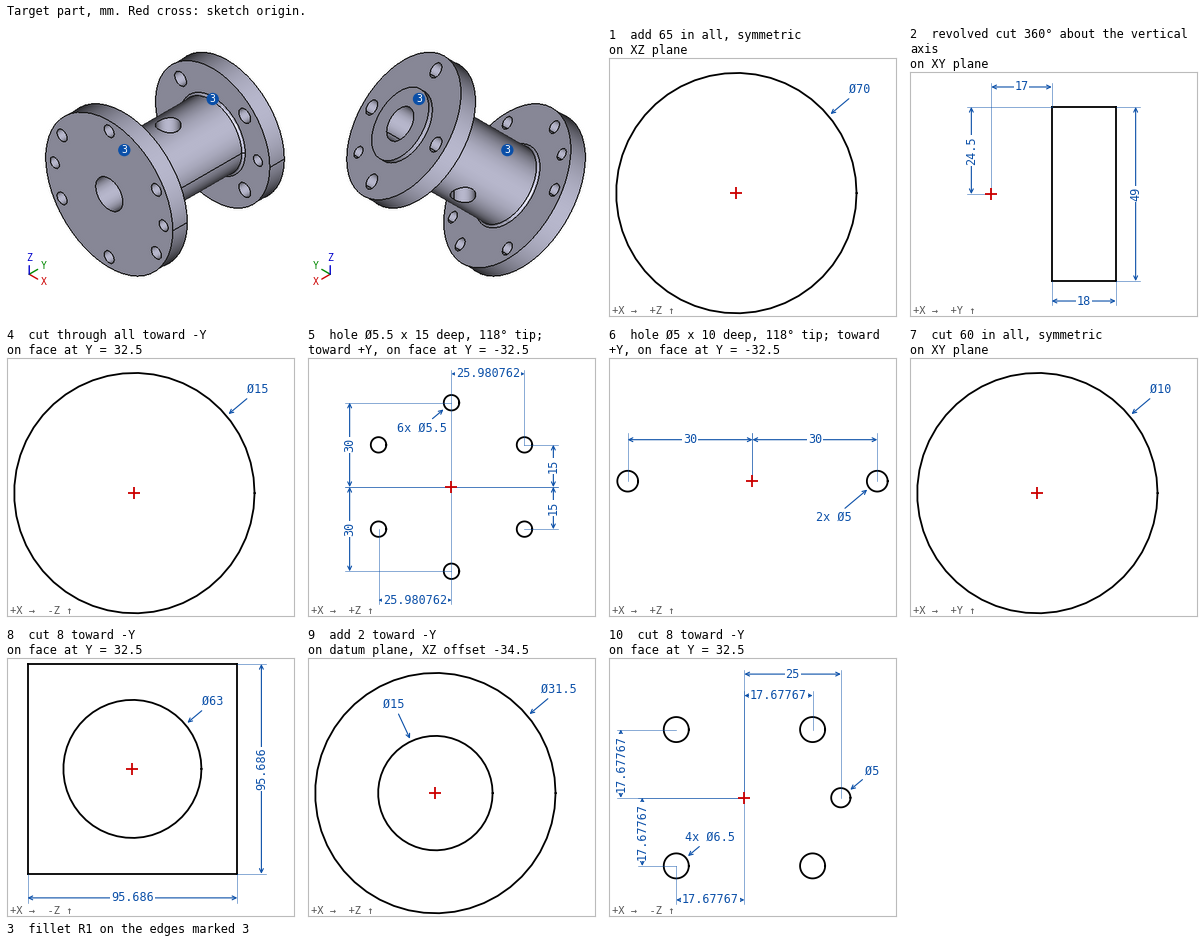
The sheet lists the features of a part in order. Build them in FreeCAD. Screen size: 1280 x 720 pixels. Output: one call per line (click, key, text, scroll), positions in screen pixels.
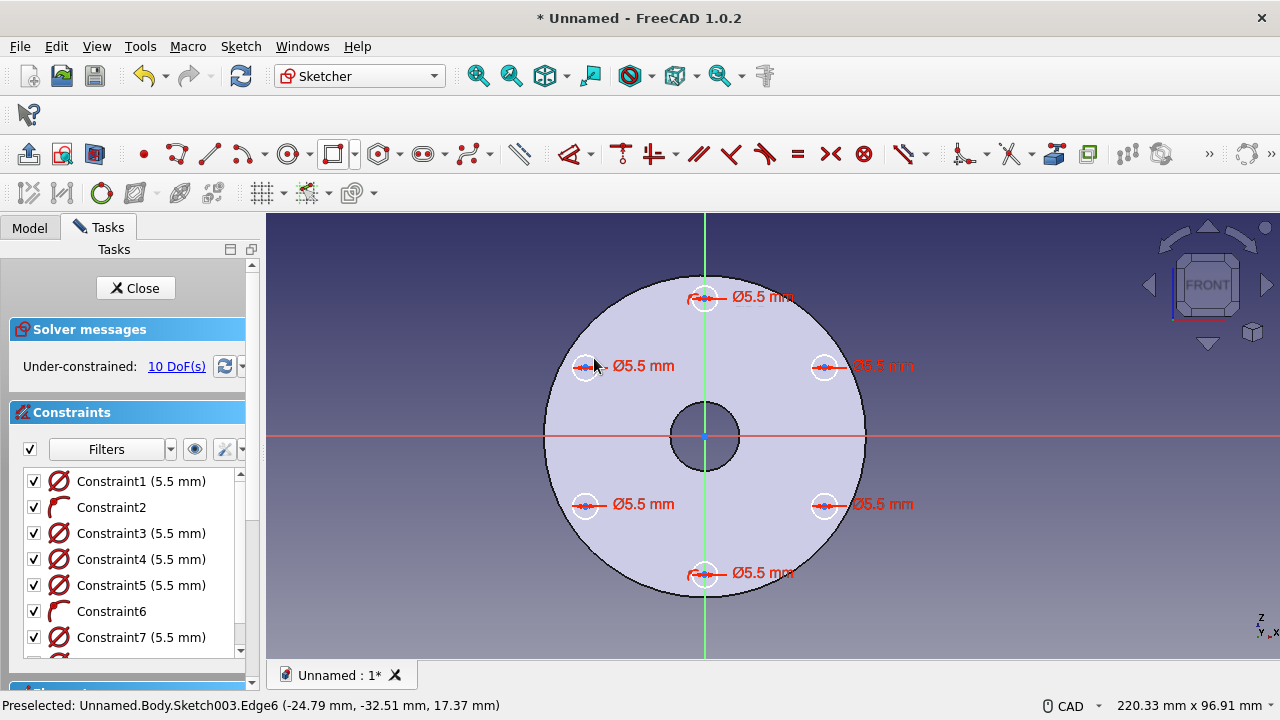
click(825, 368)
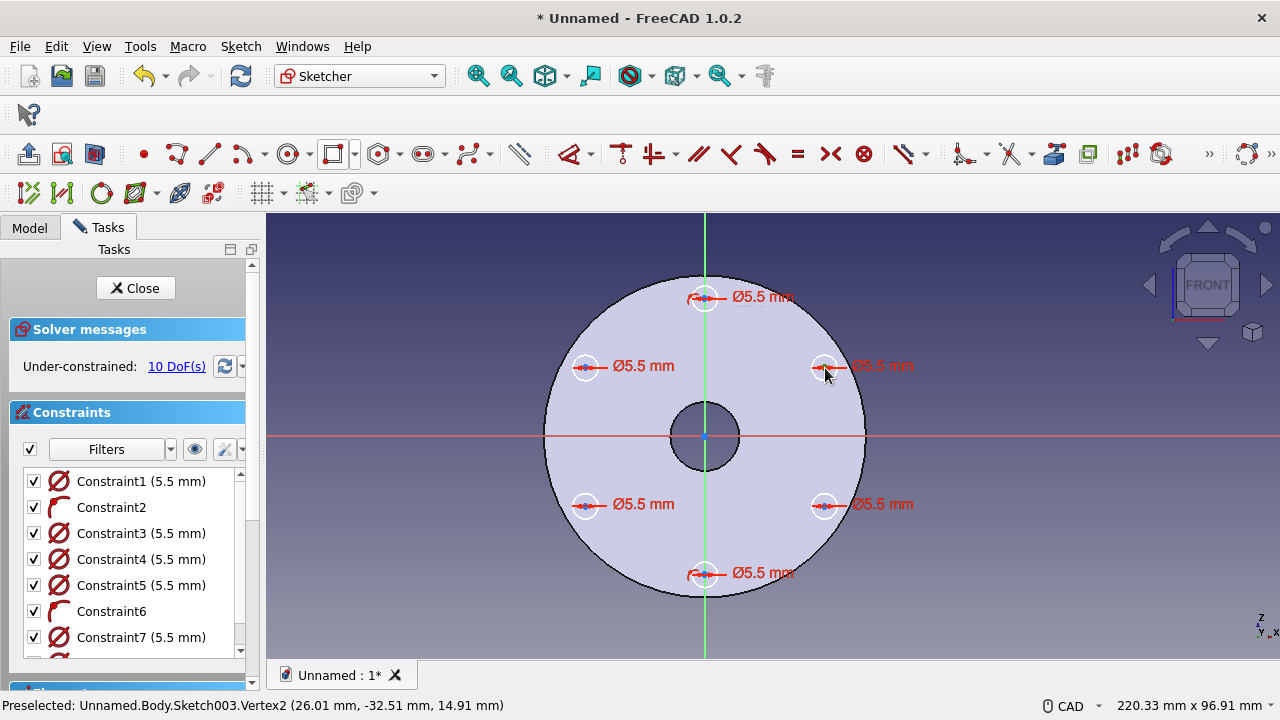
click(825, 506)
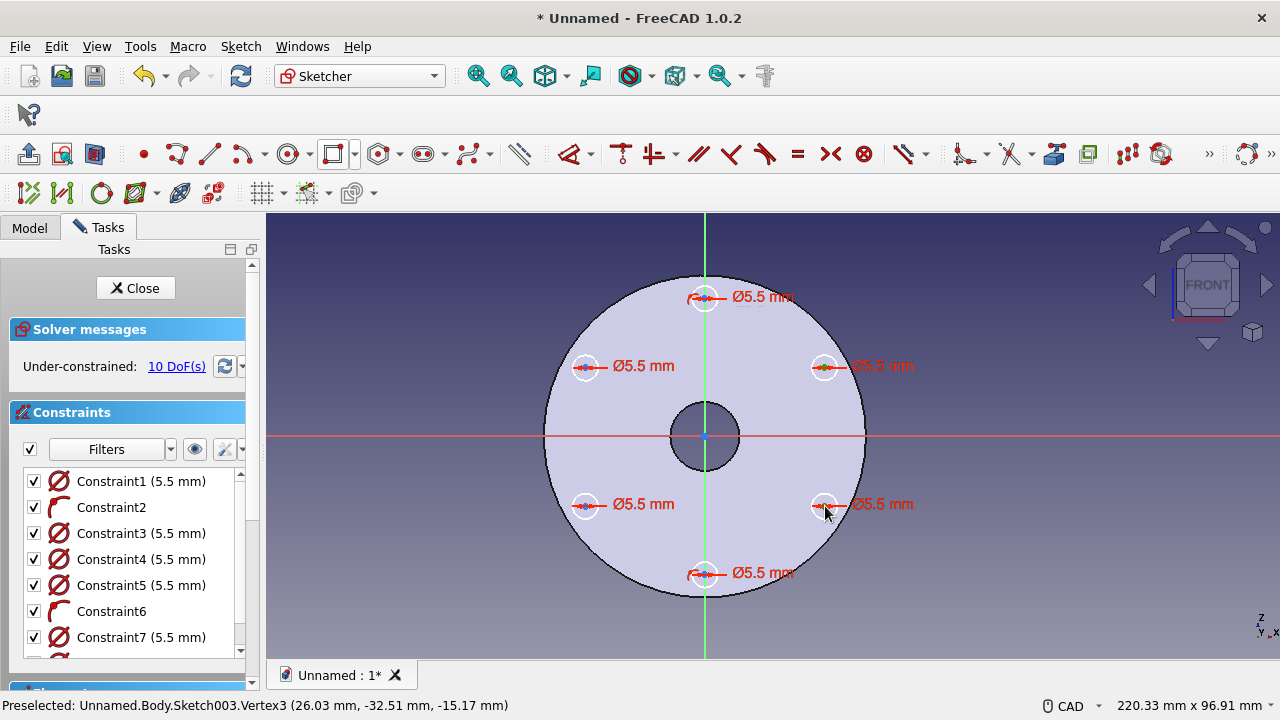
click(676, 154)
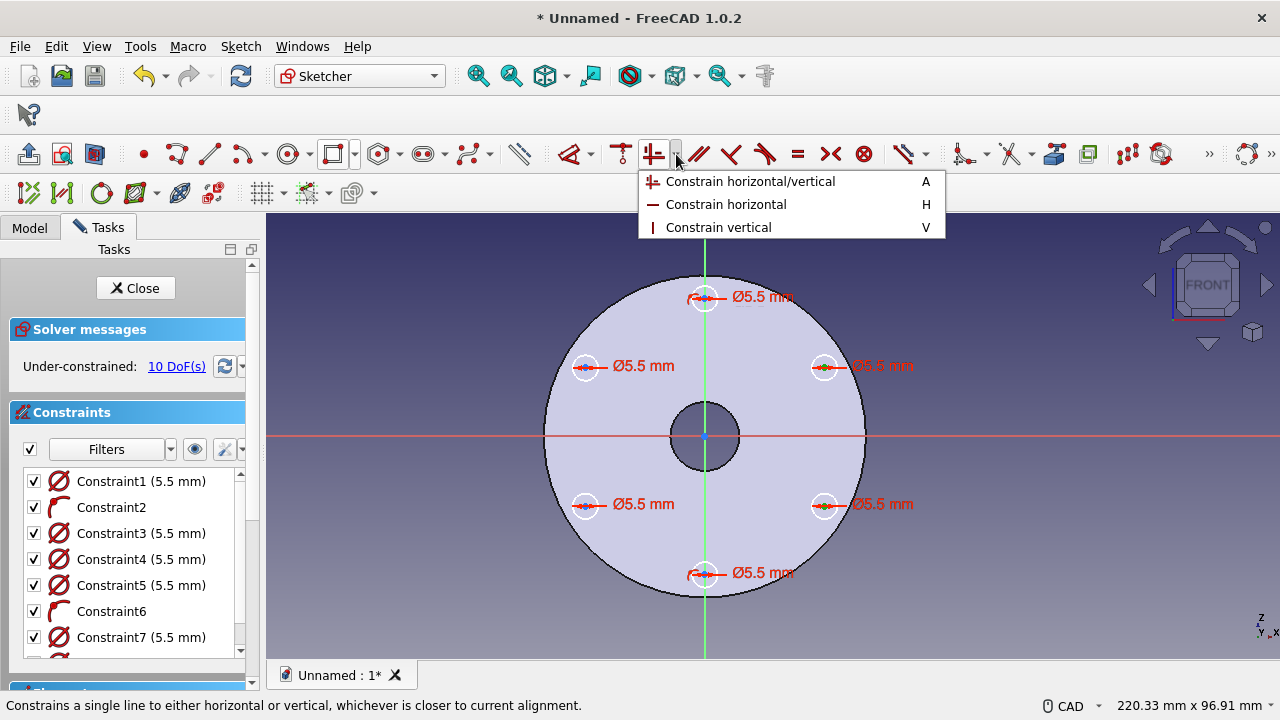
click(792, 228)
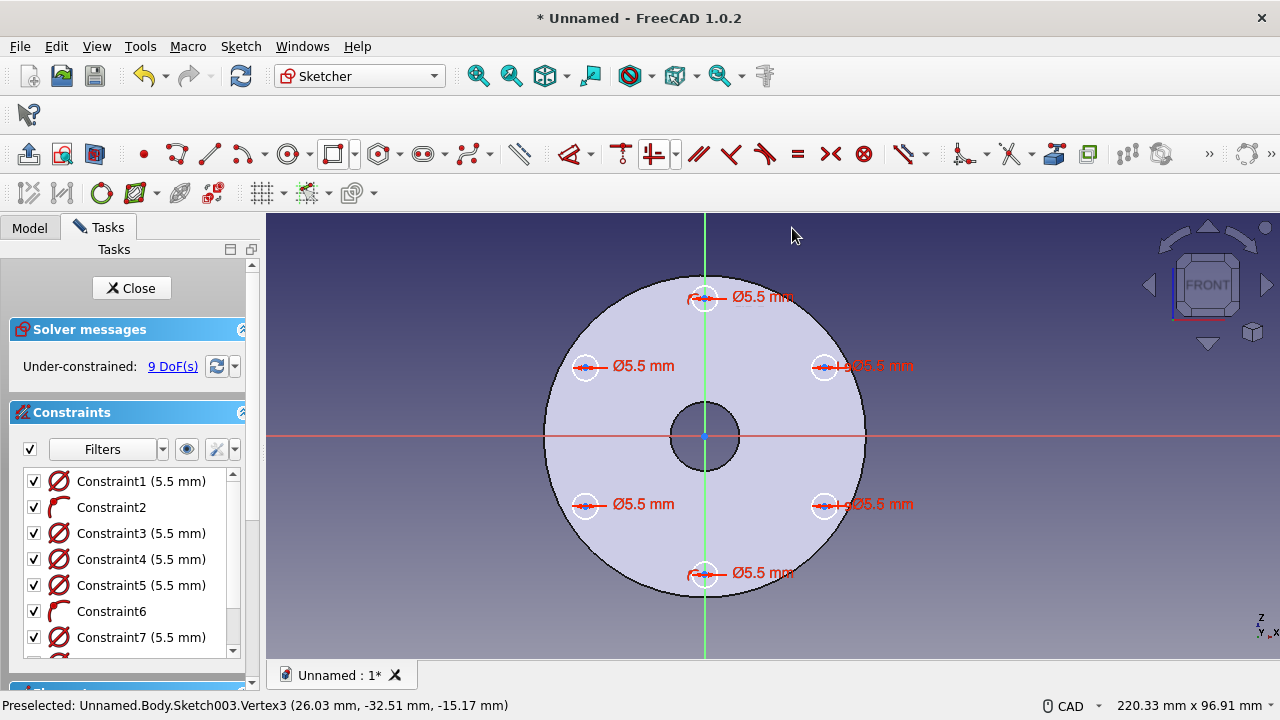
click(825, 506)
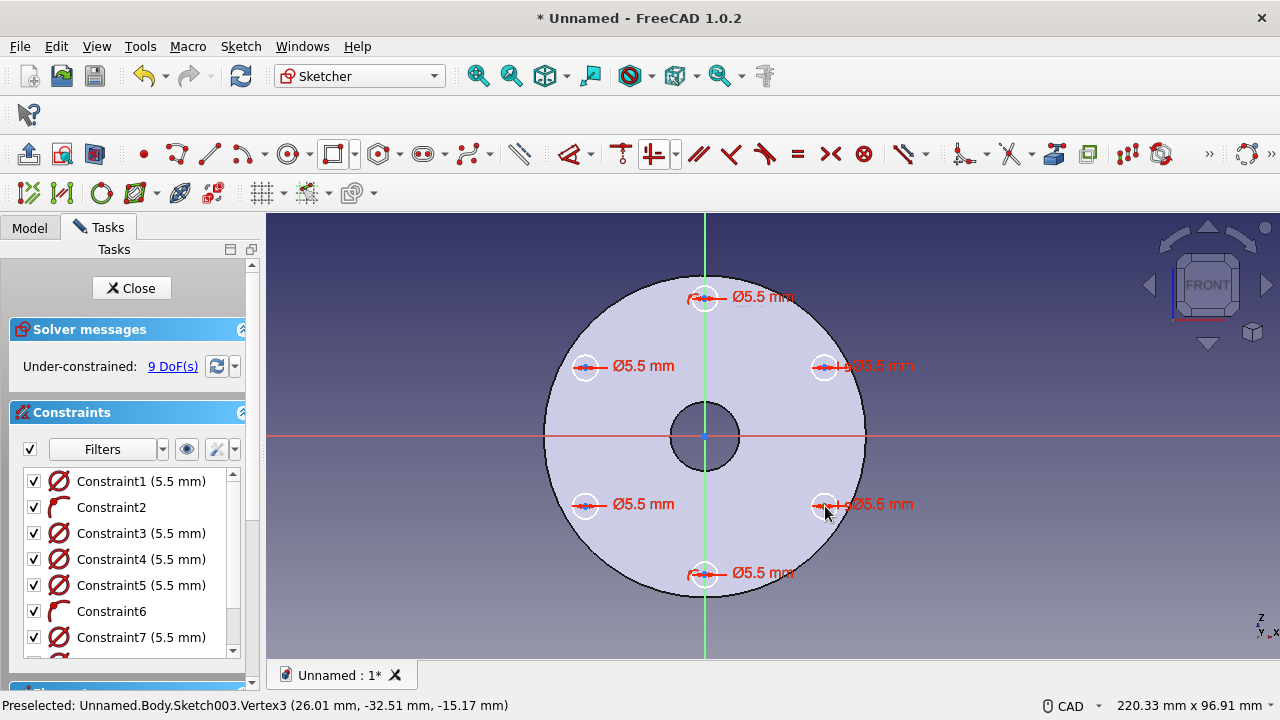
click(585, 506)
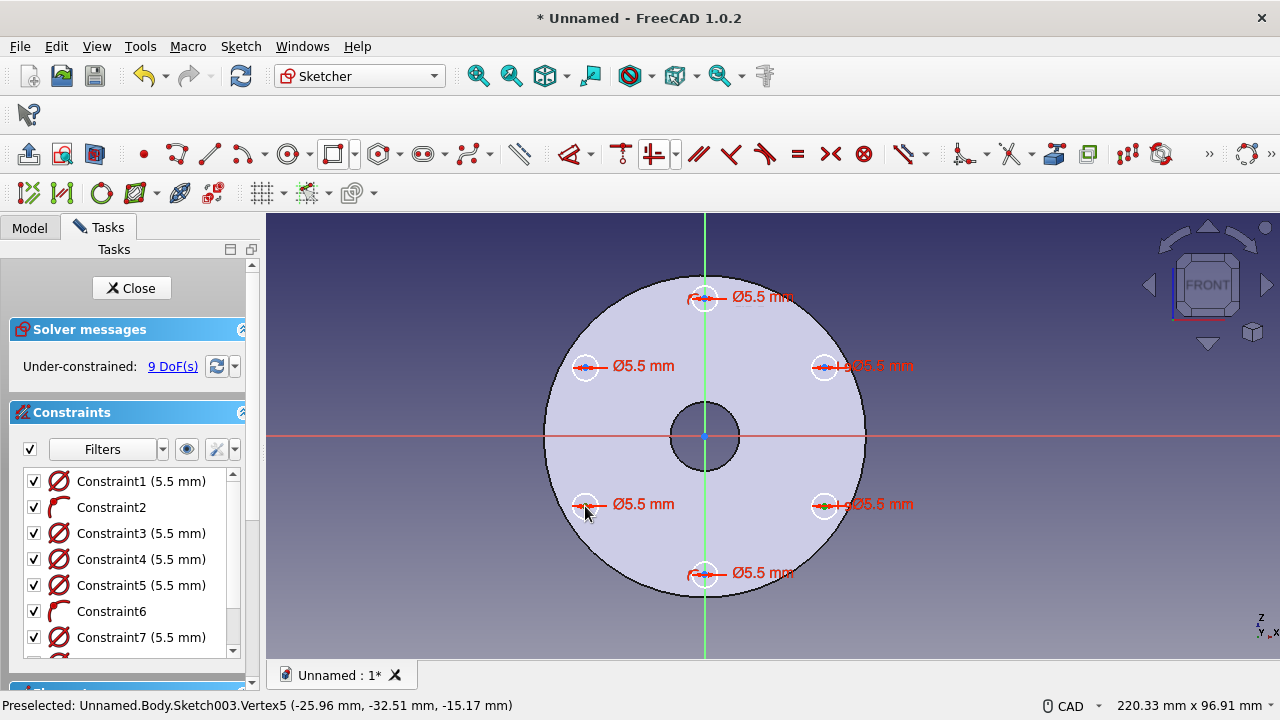
click(676, 154)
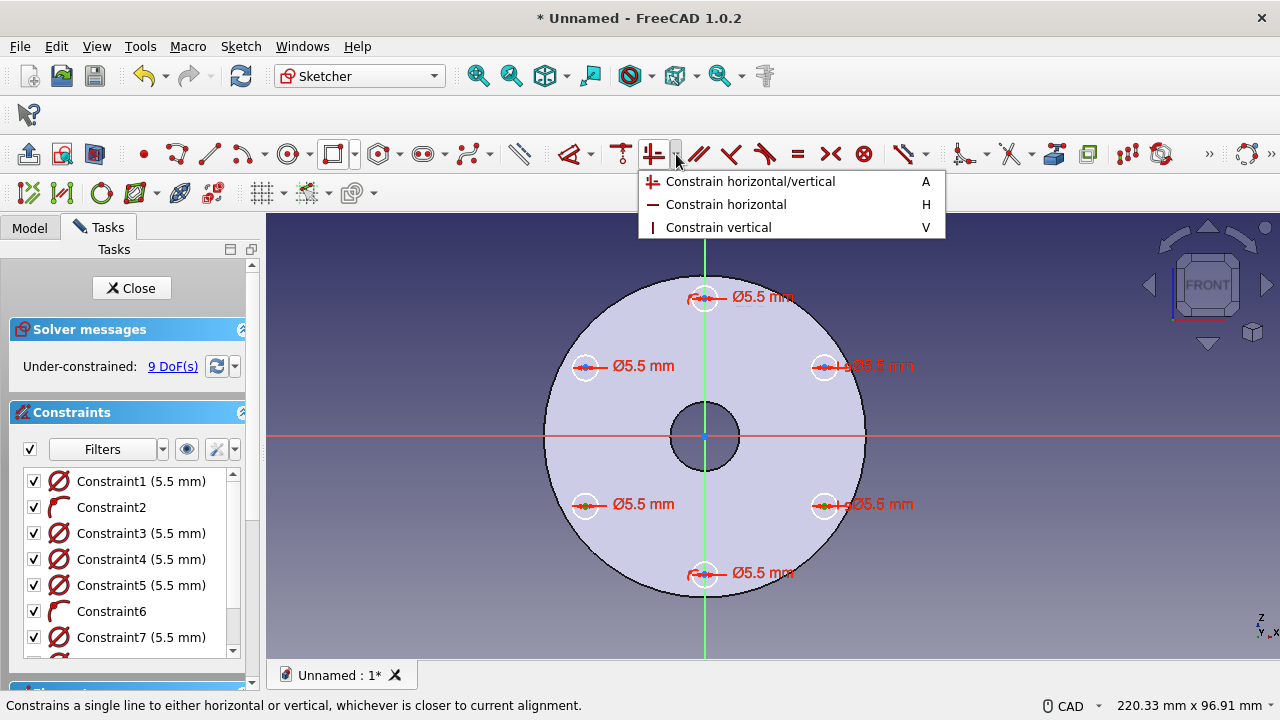
click(792, 204)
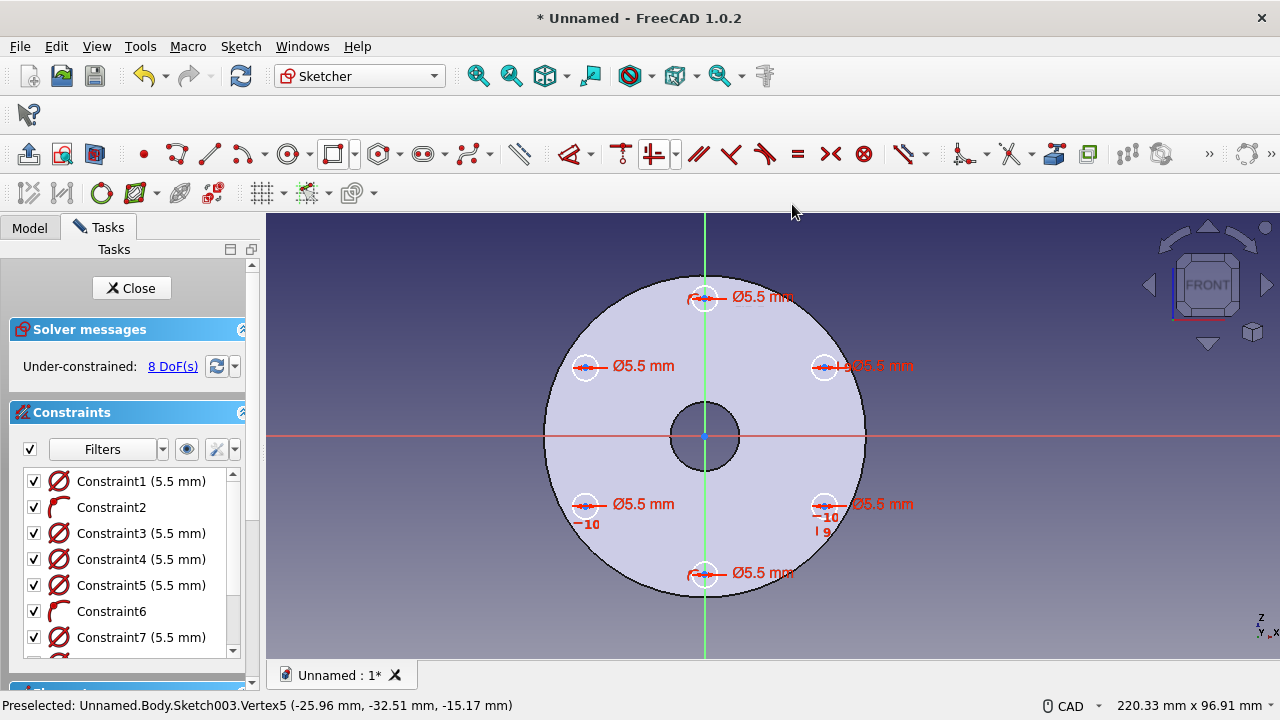
click(585, 506)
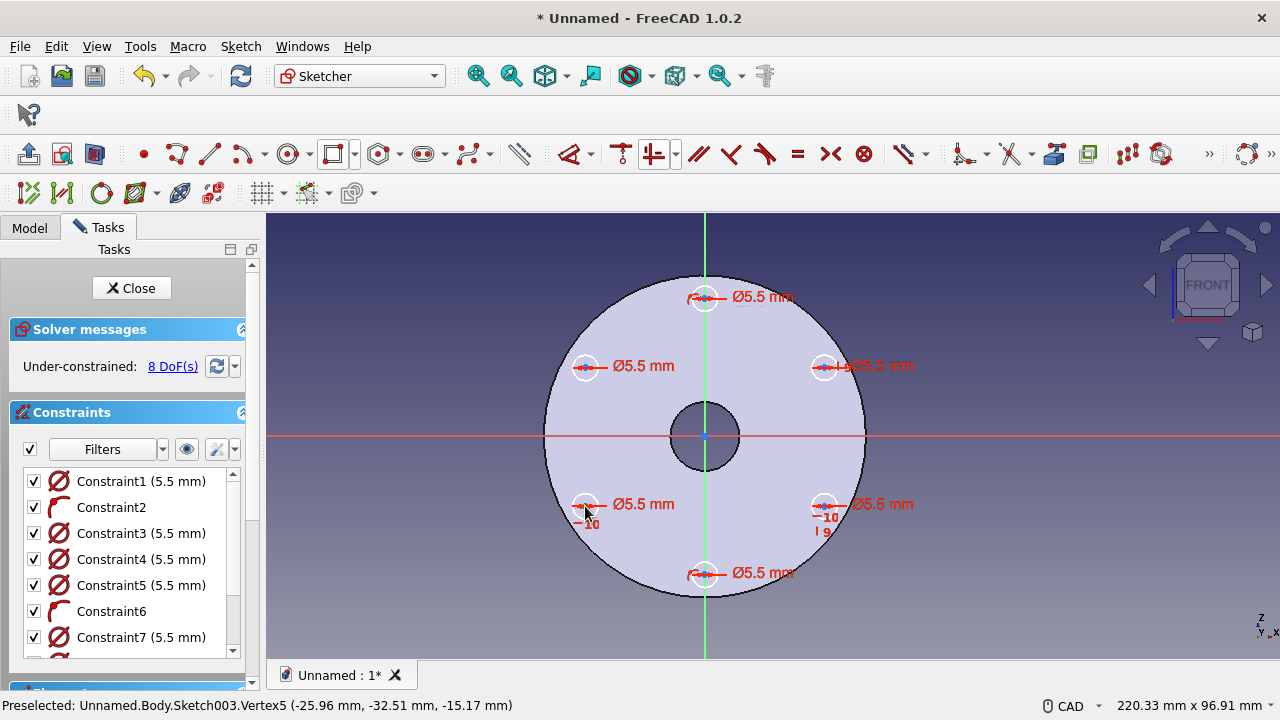
click(585, 368)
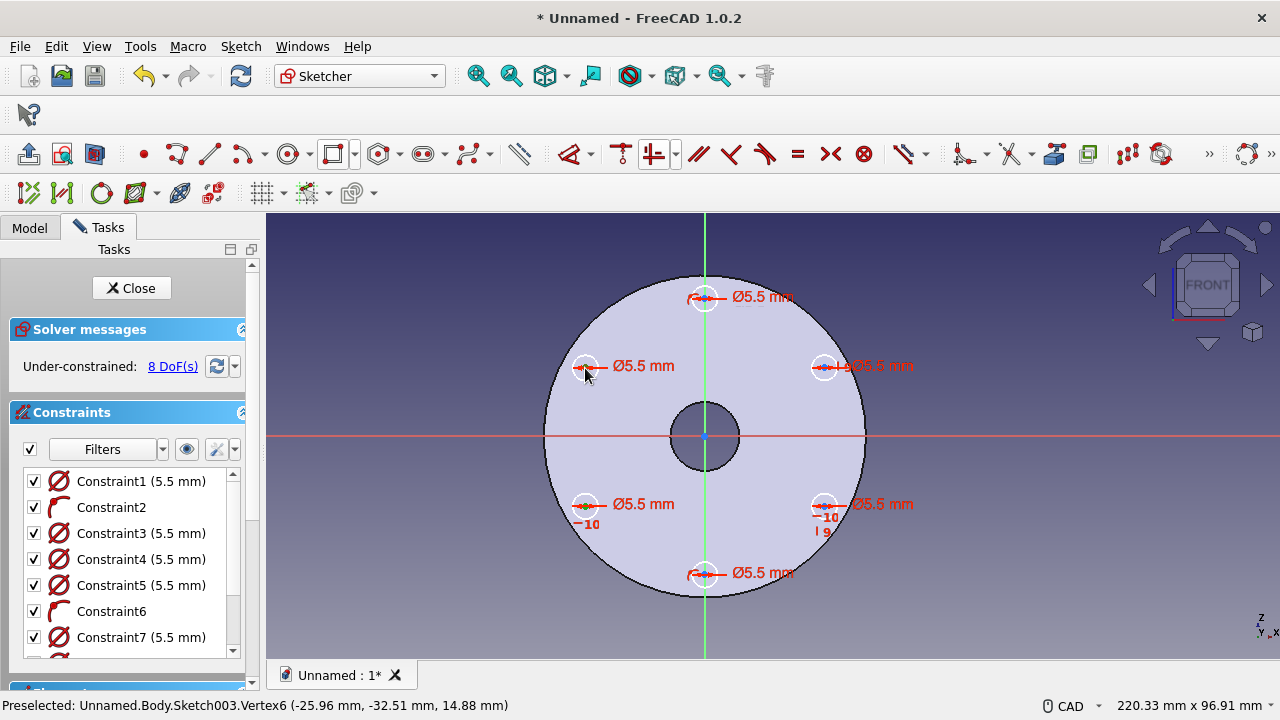
key(v)